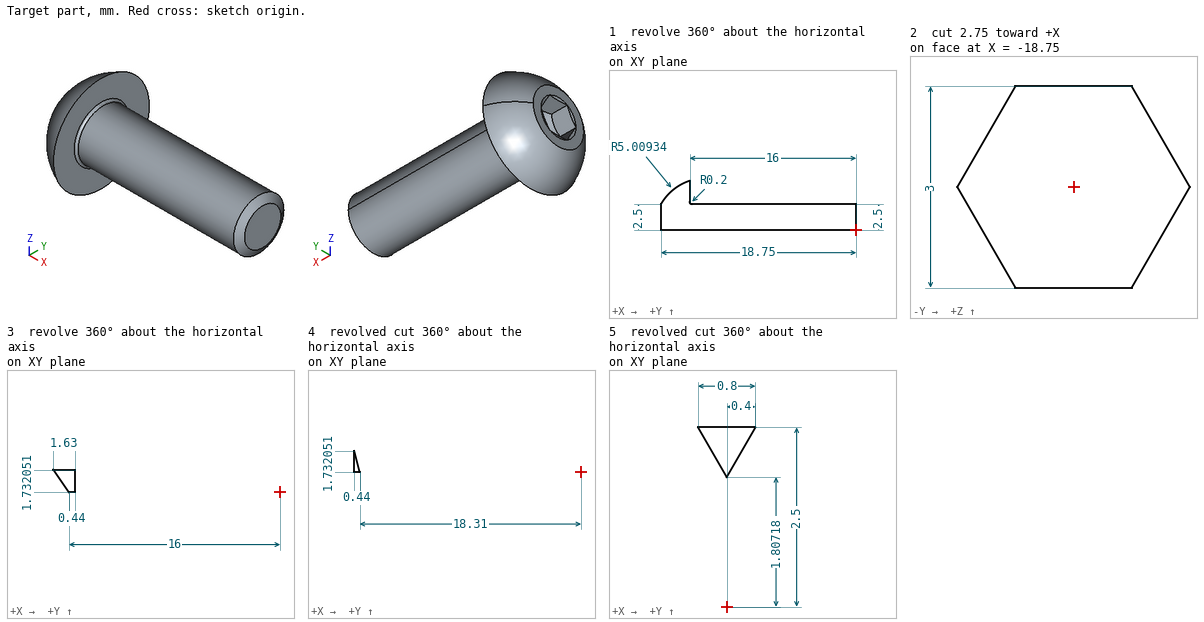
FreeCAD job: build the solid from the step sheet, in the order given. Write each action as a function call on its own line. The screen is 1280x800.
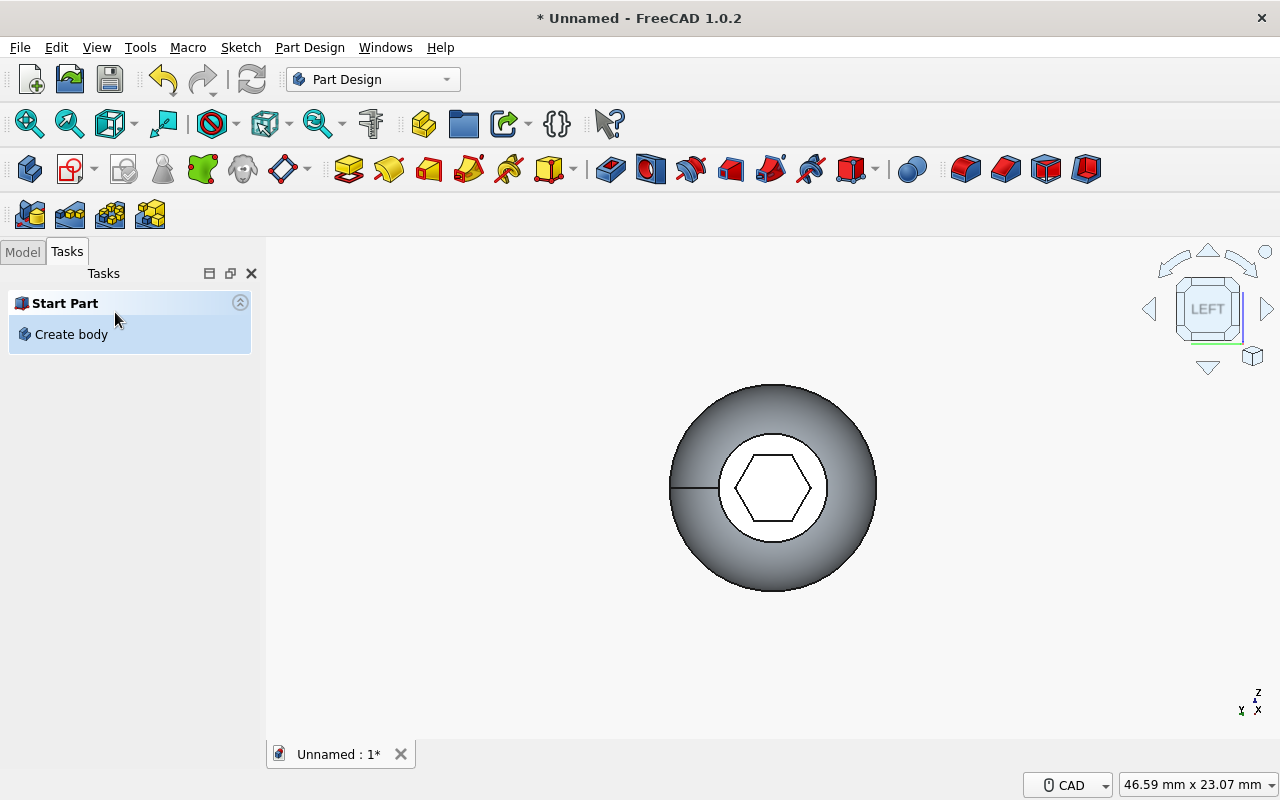
click(30, 124)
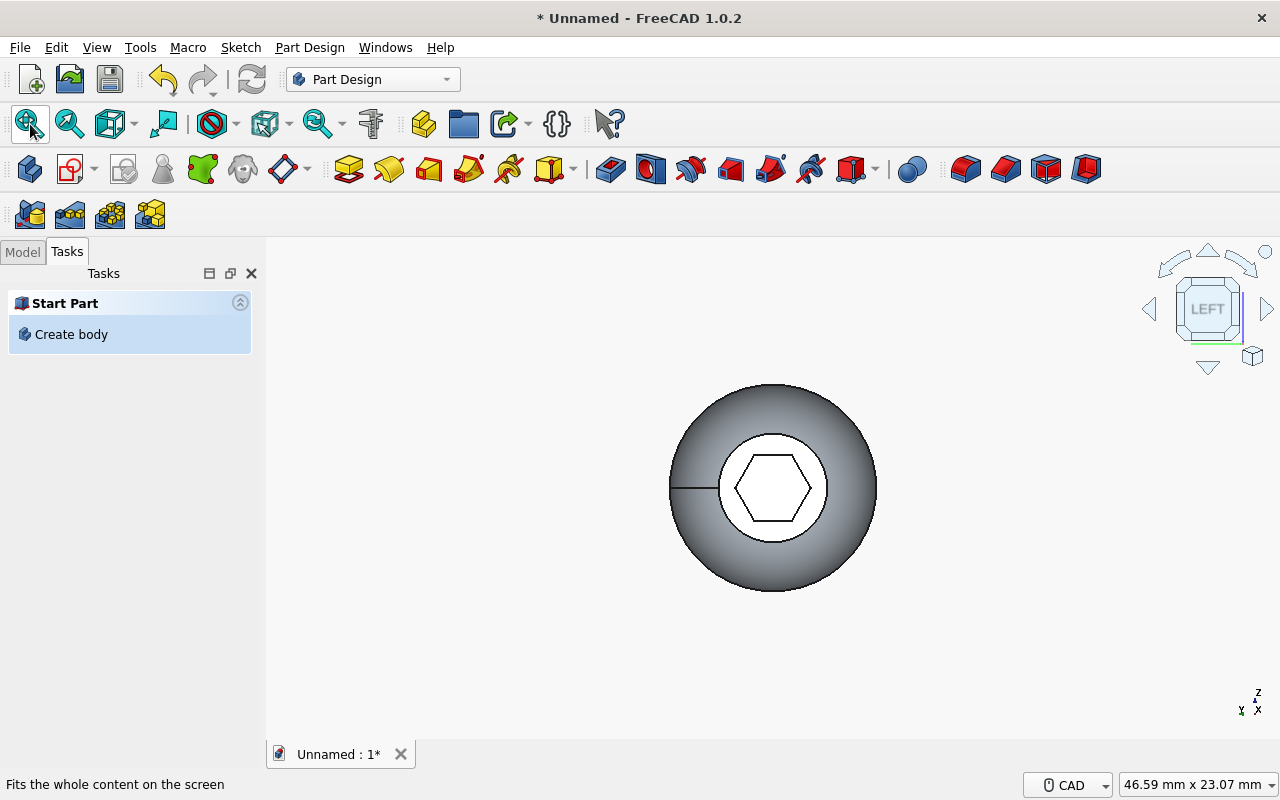
click(70, 170)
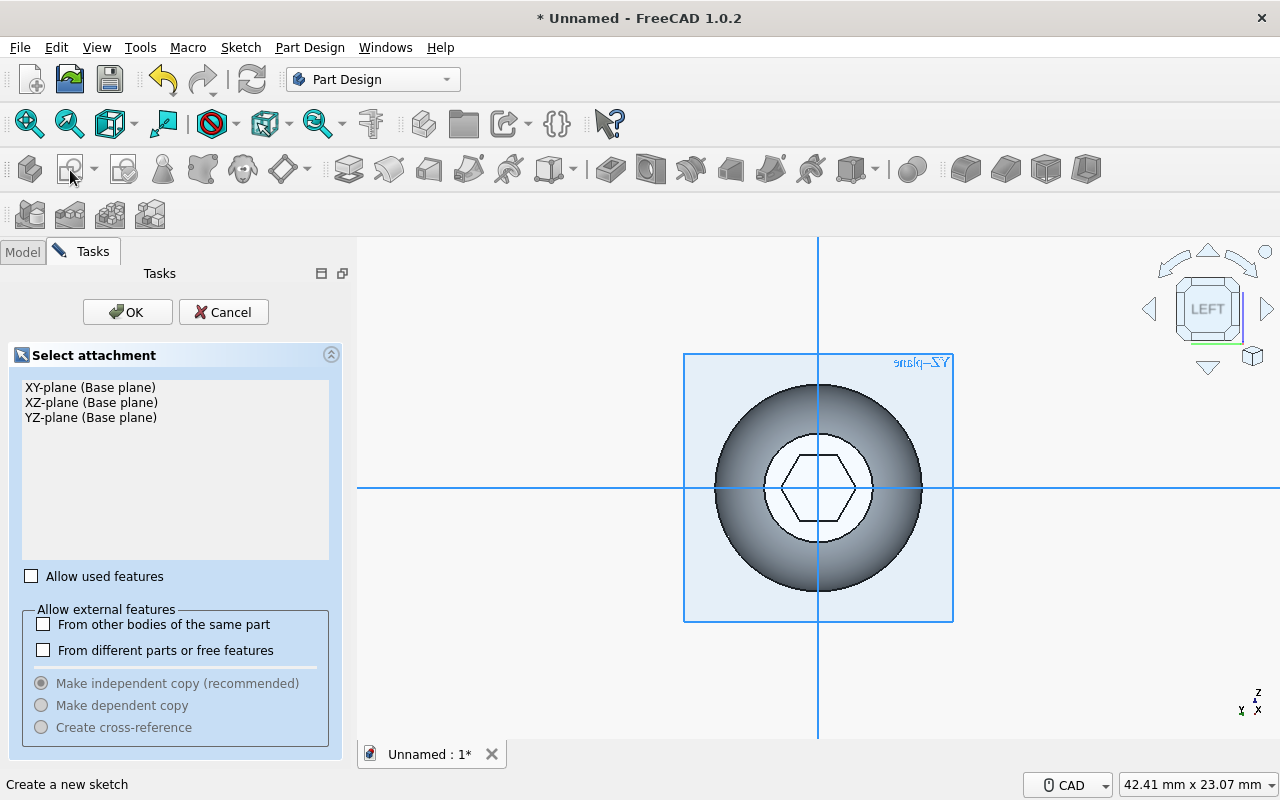
click(82, 388)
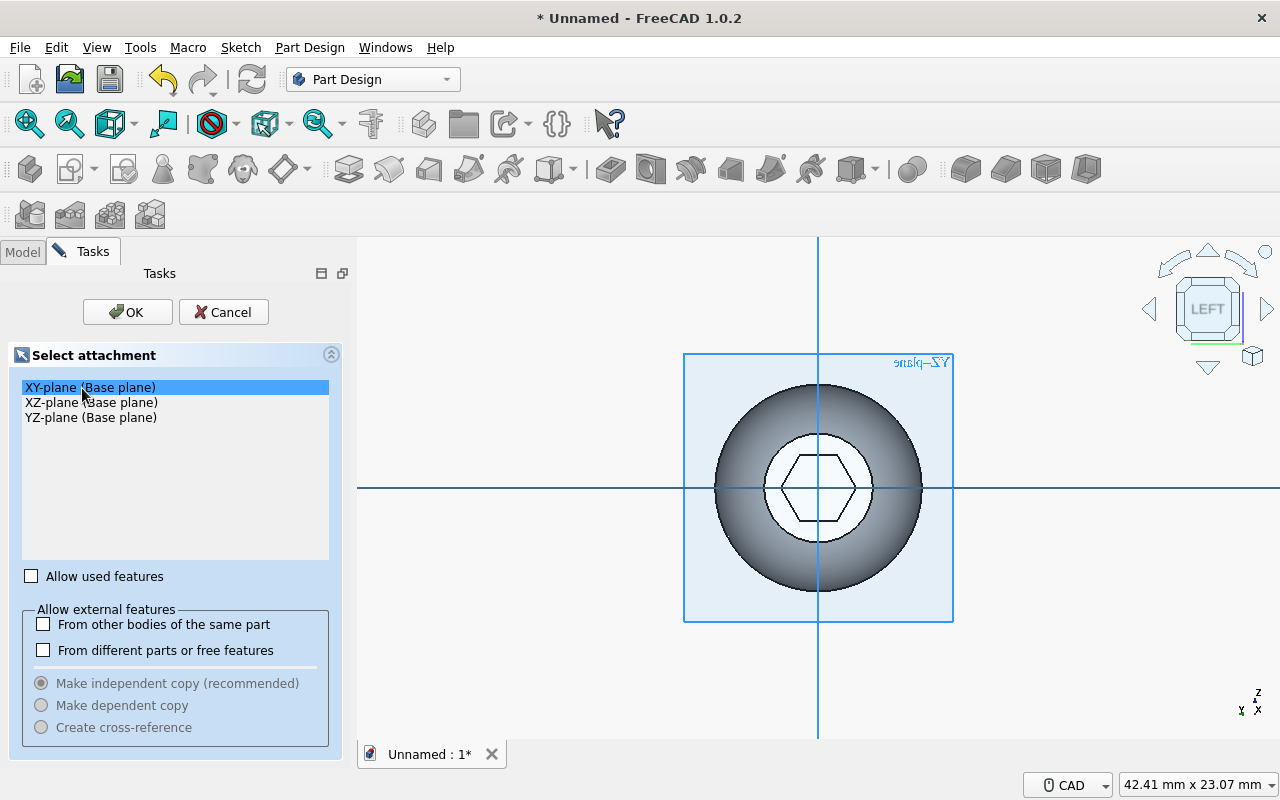
click(128, 312)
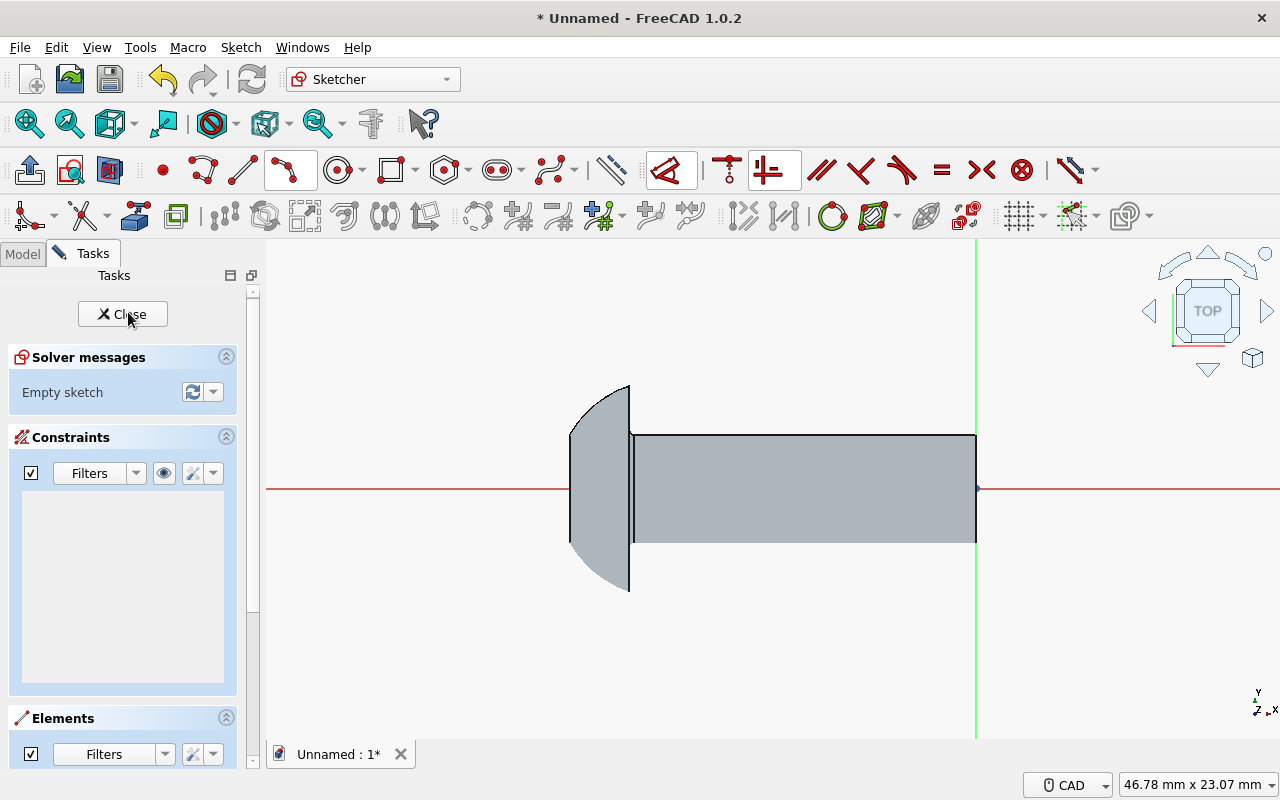
click(110, 170)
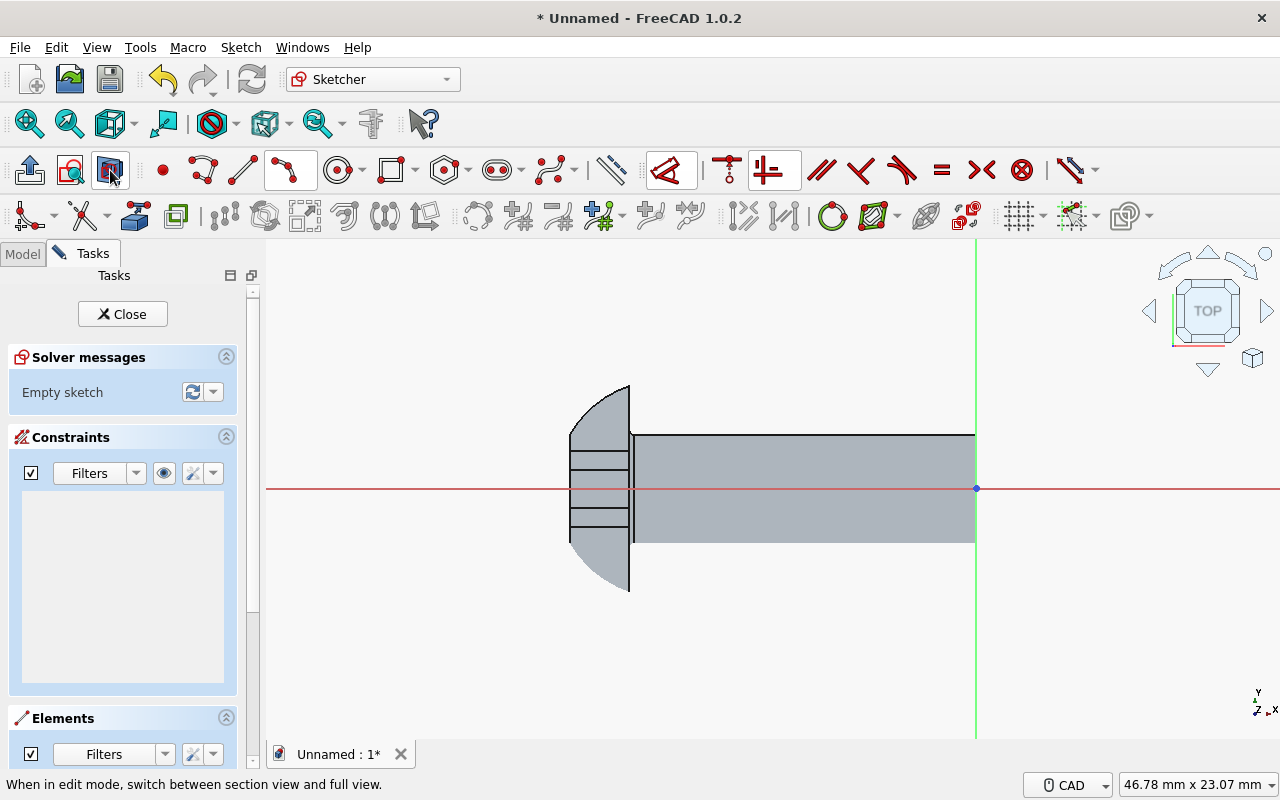
scroll(611, 468, up, 11)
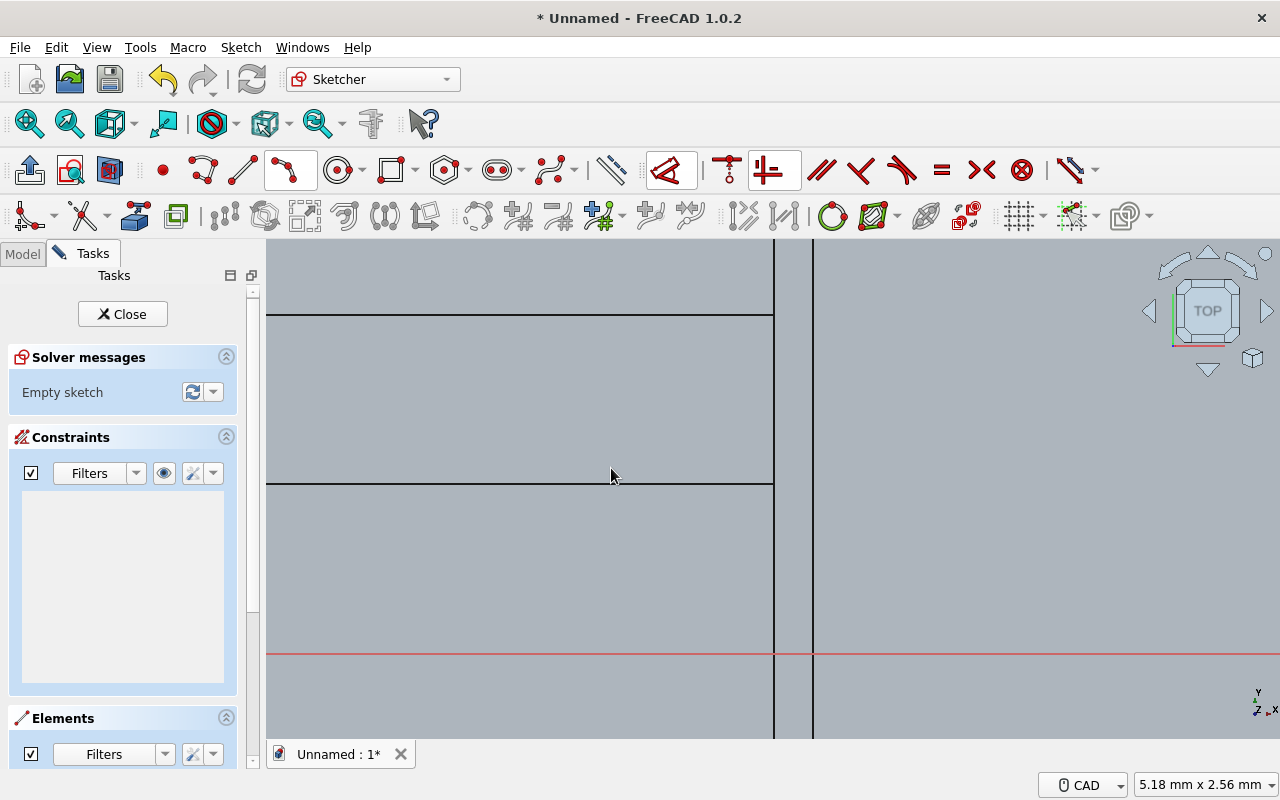
click(204, 170)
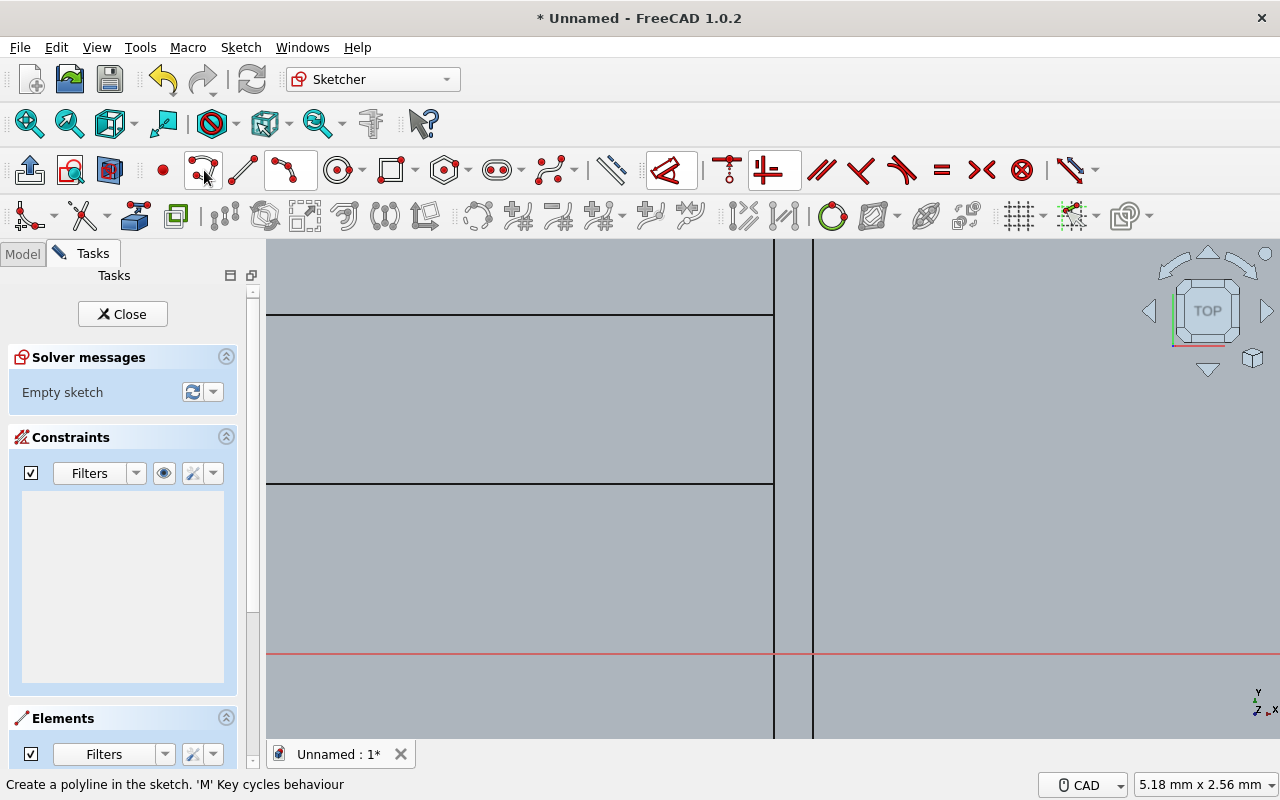
click(860, 654)
click(860, 315)
click(541, 315)
click(774, 645)
click(860, 654)
key(Escape)
key(Escape)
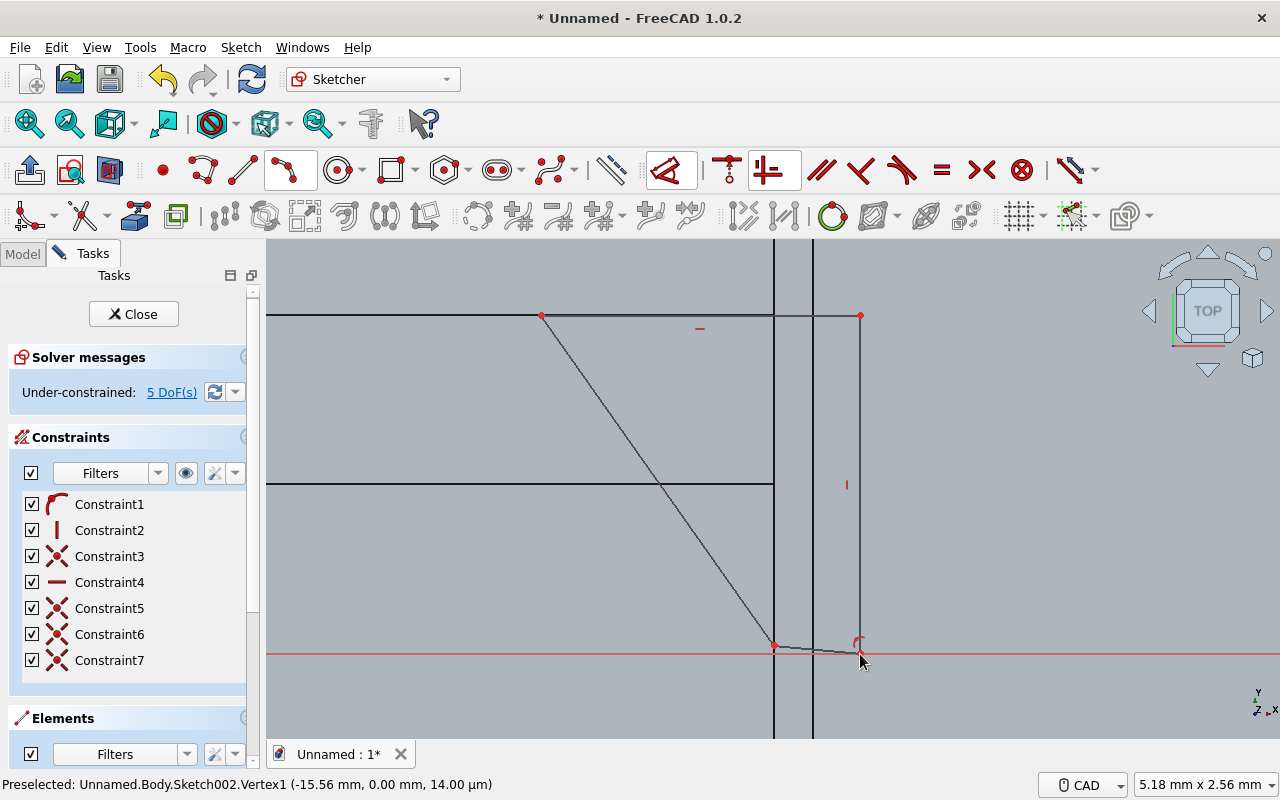
click(834, 651)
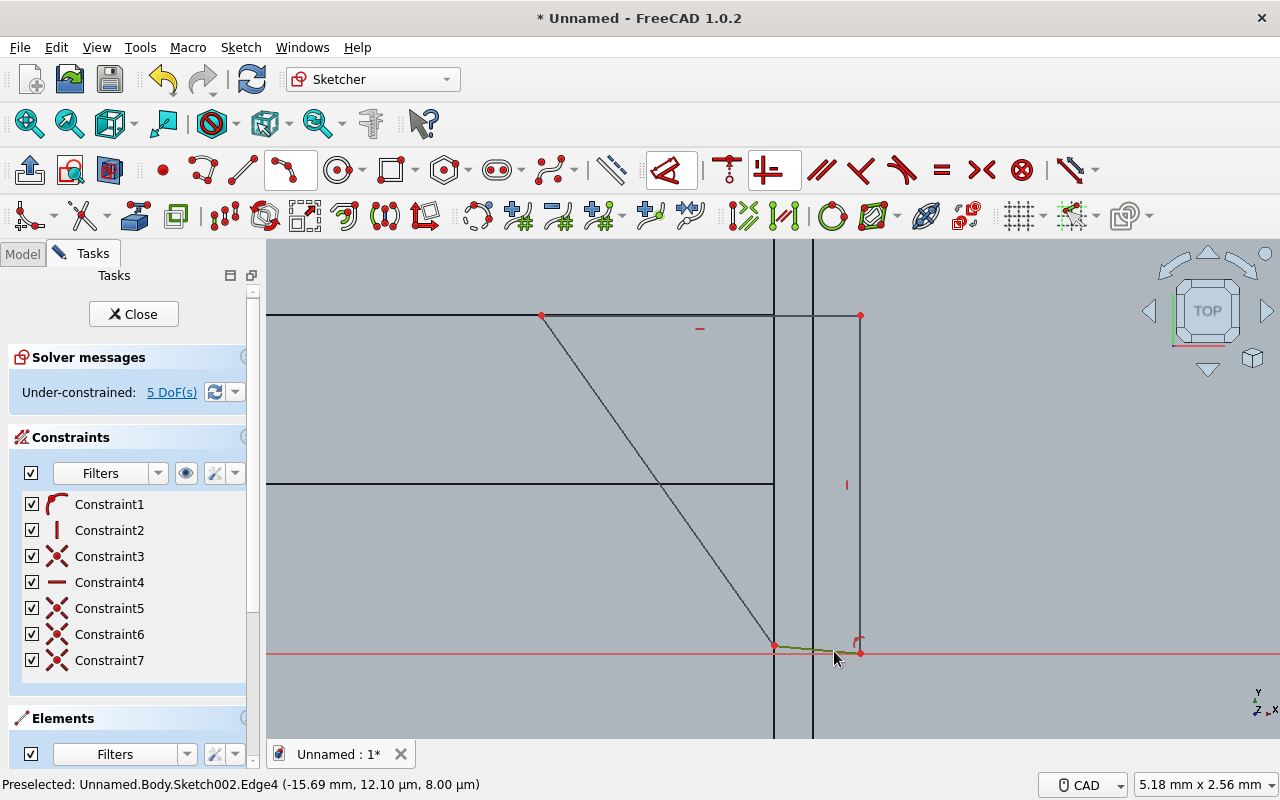
key(h)